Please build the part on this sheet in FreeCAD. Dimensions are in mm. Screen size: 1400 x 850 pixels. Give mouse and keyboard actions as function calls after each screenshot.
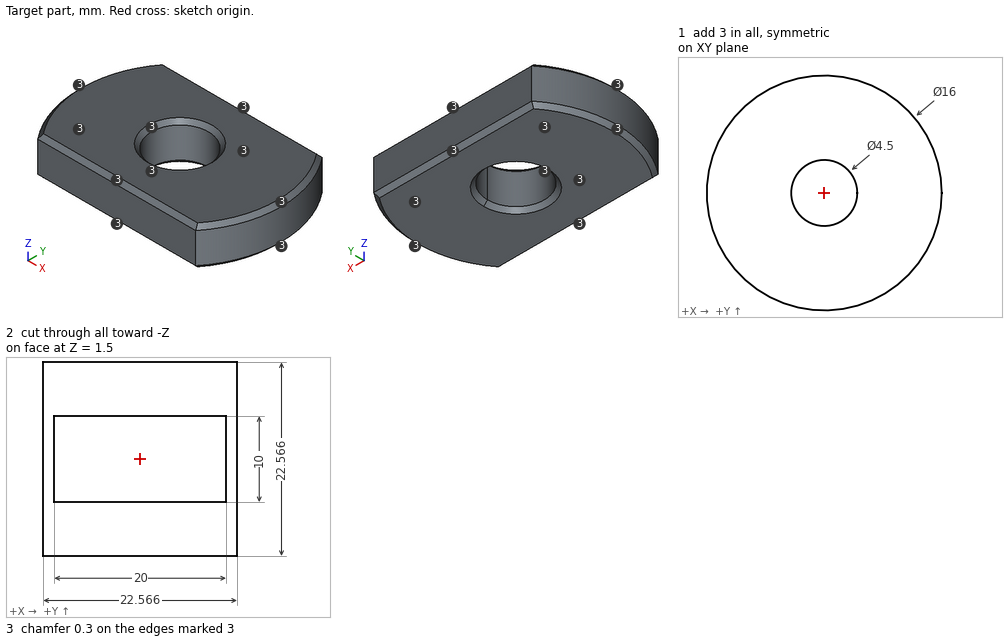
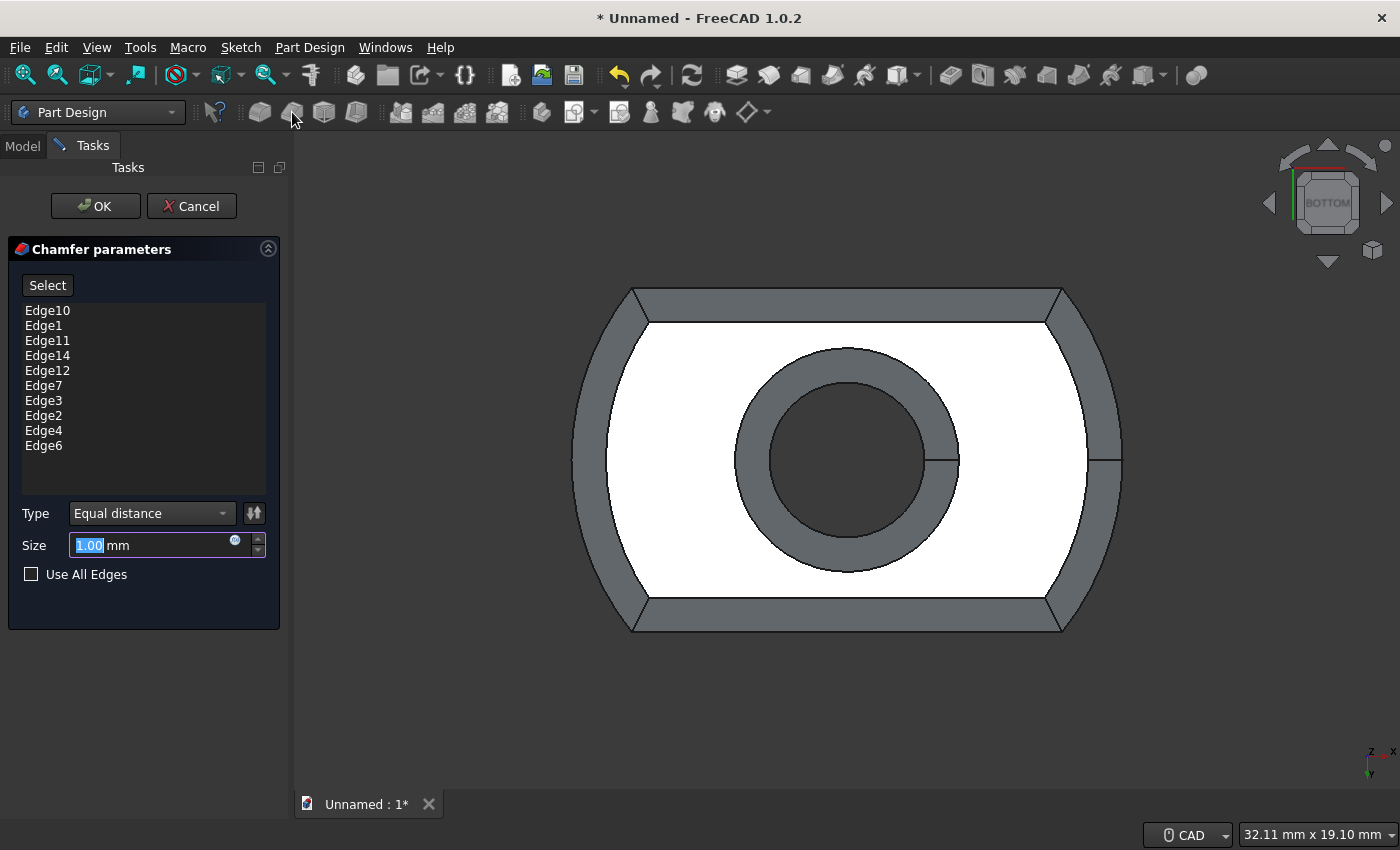
text(0.3)
key(Tab)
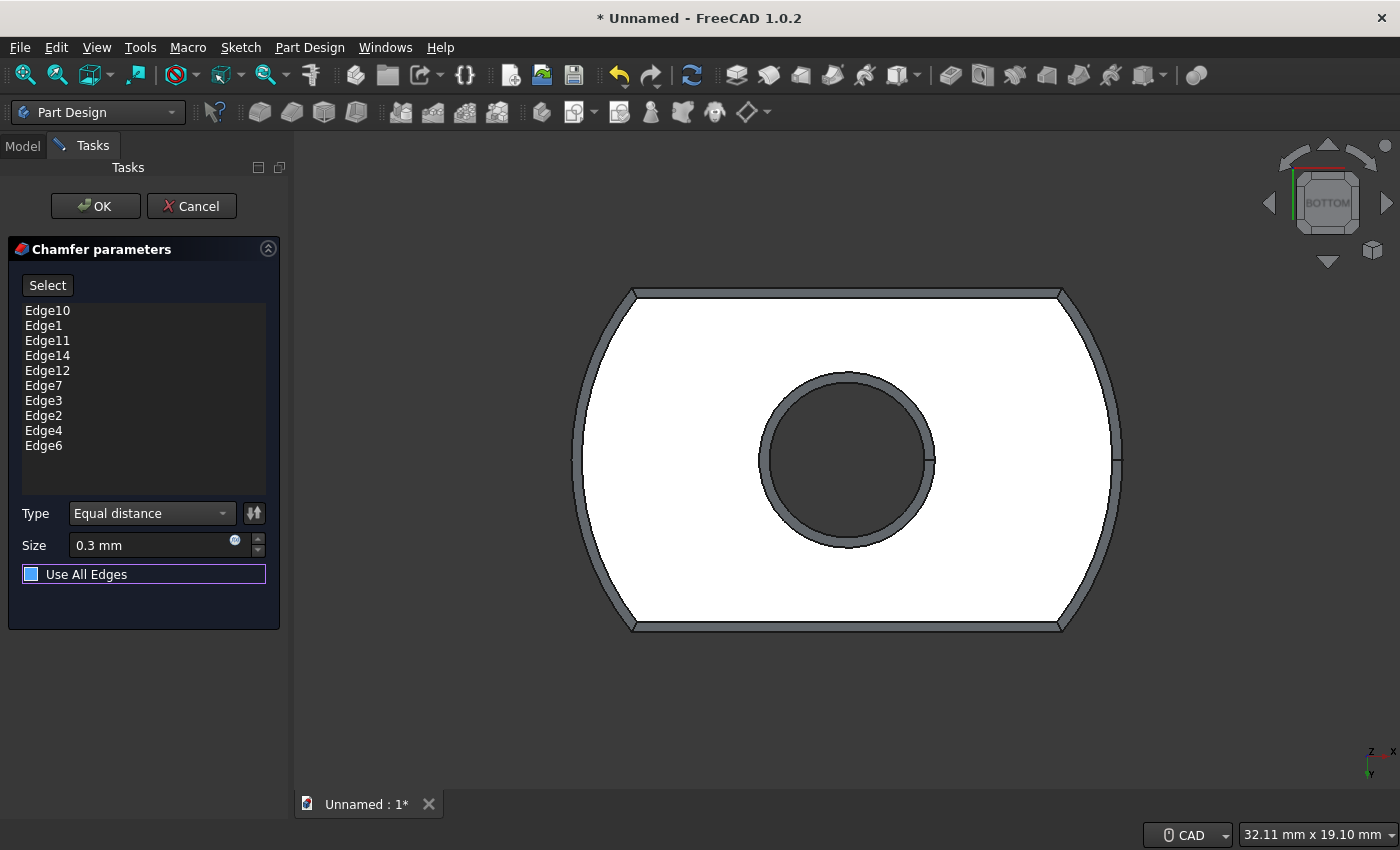
click(96, 206)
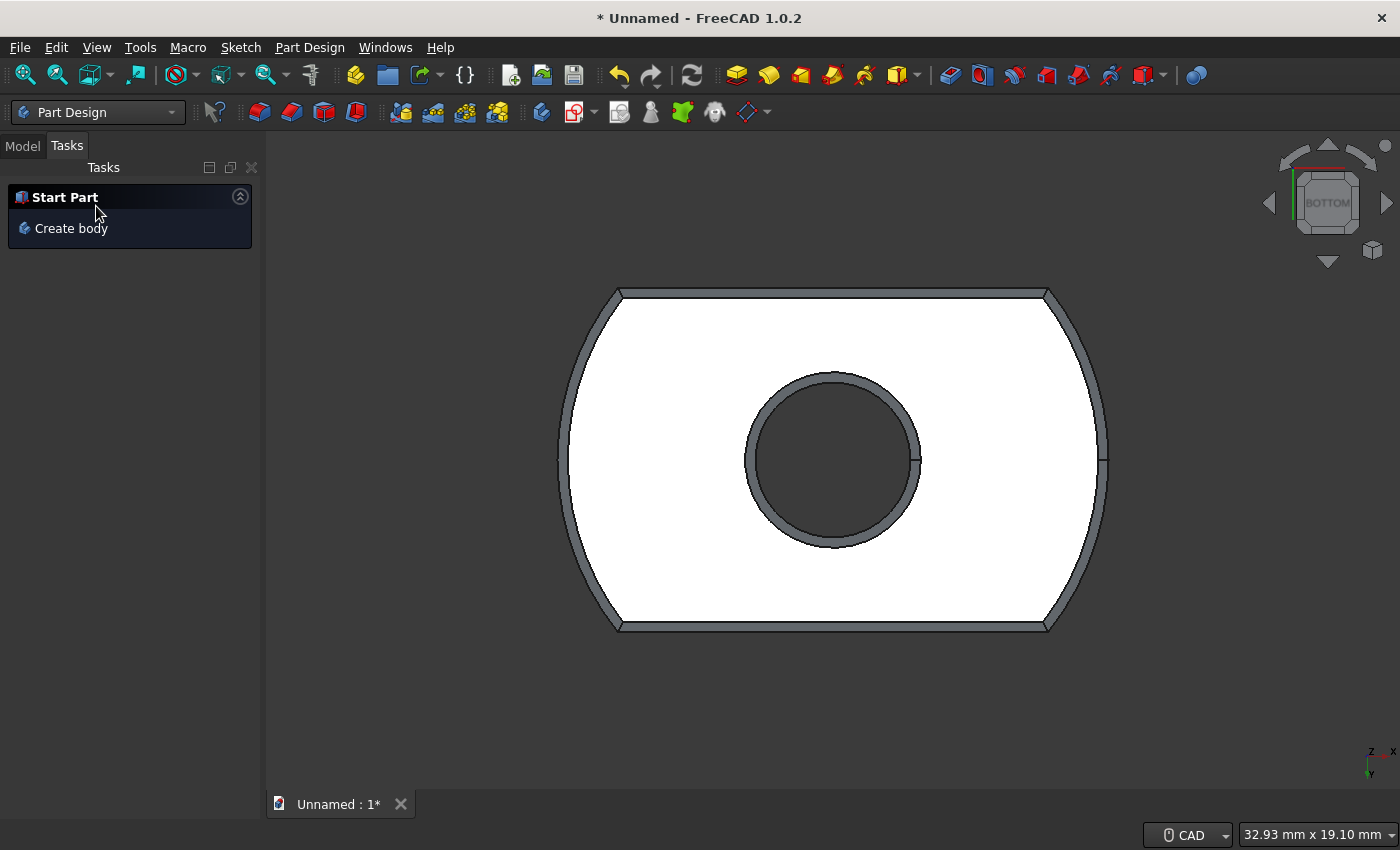
key(0)